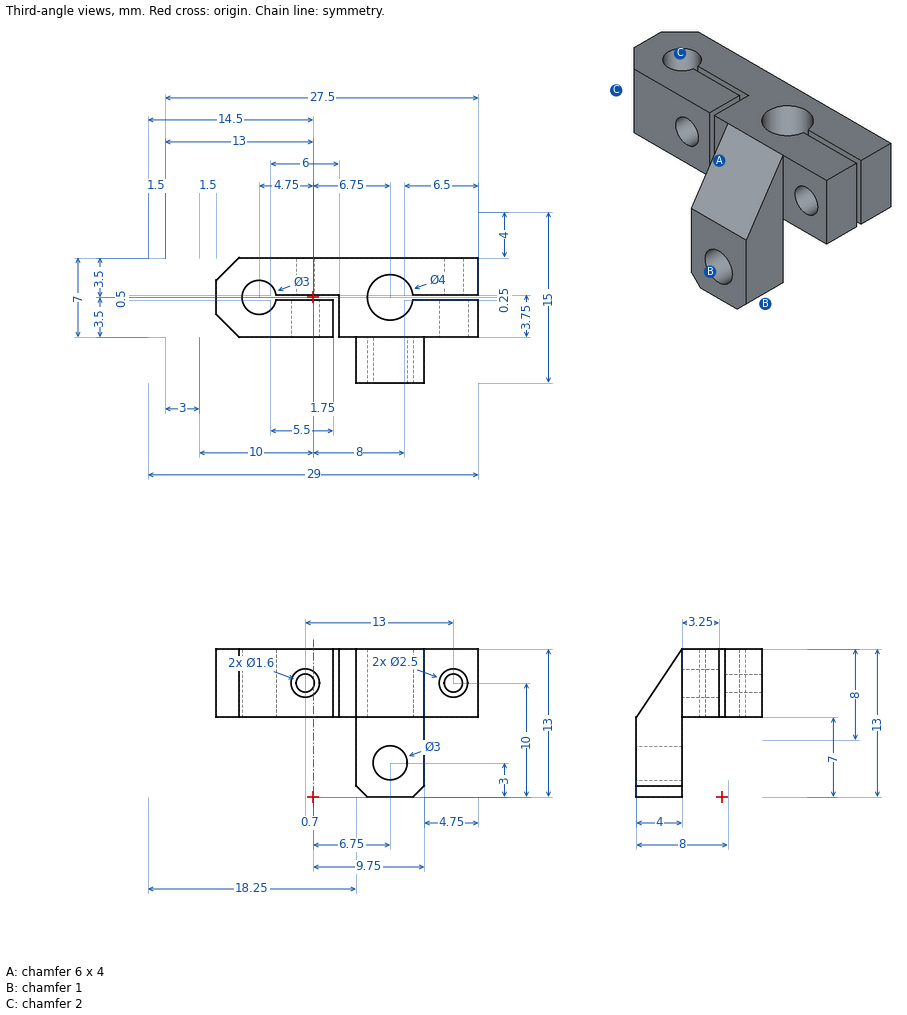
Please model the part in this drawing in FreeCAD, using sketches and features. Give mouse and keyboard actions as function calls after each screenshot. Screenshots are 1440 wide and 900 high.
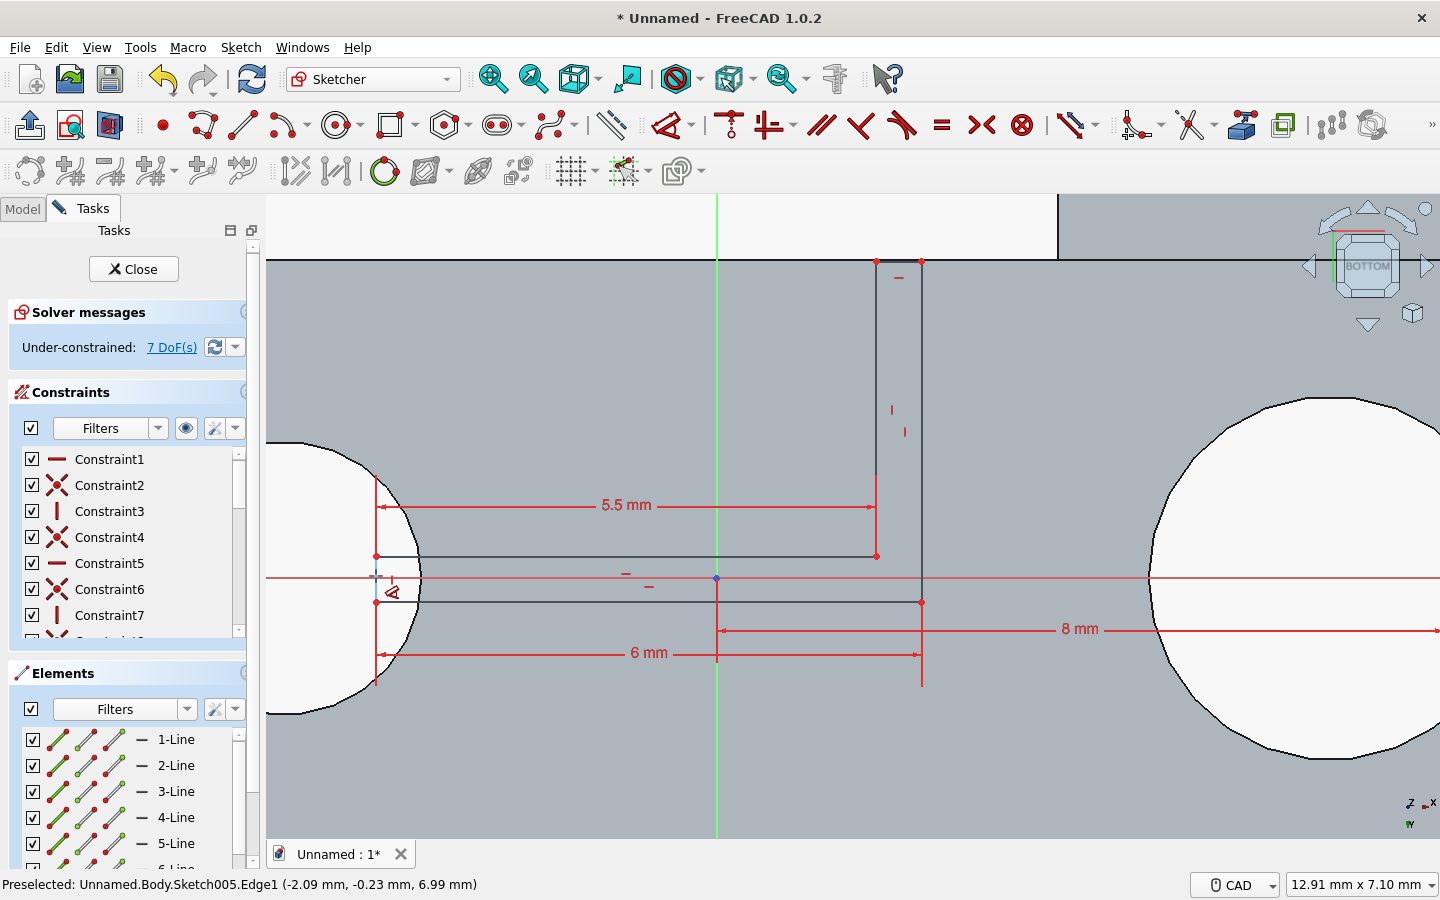
click(376, 575)
click(342, 564)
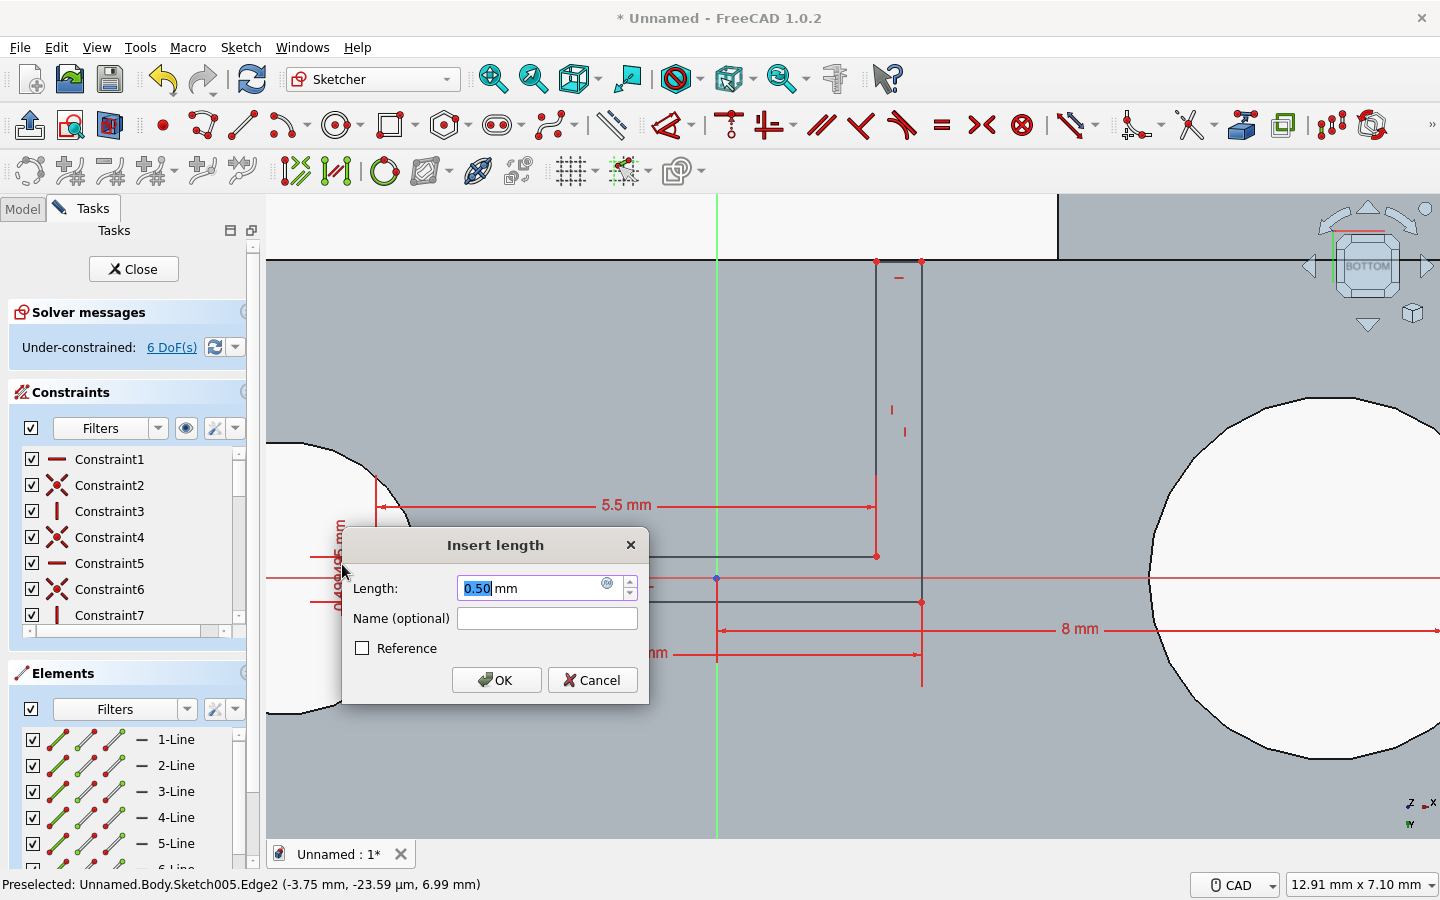
text(0.5)
key(Return)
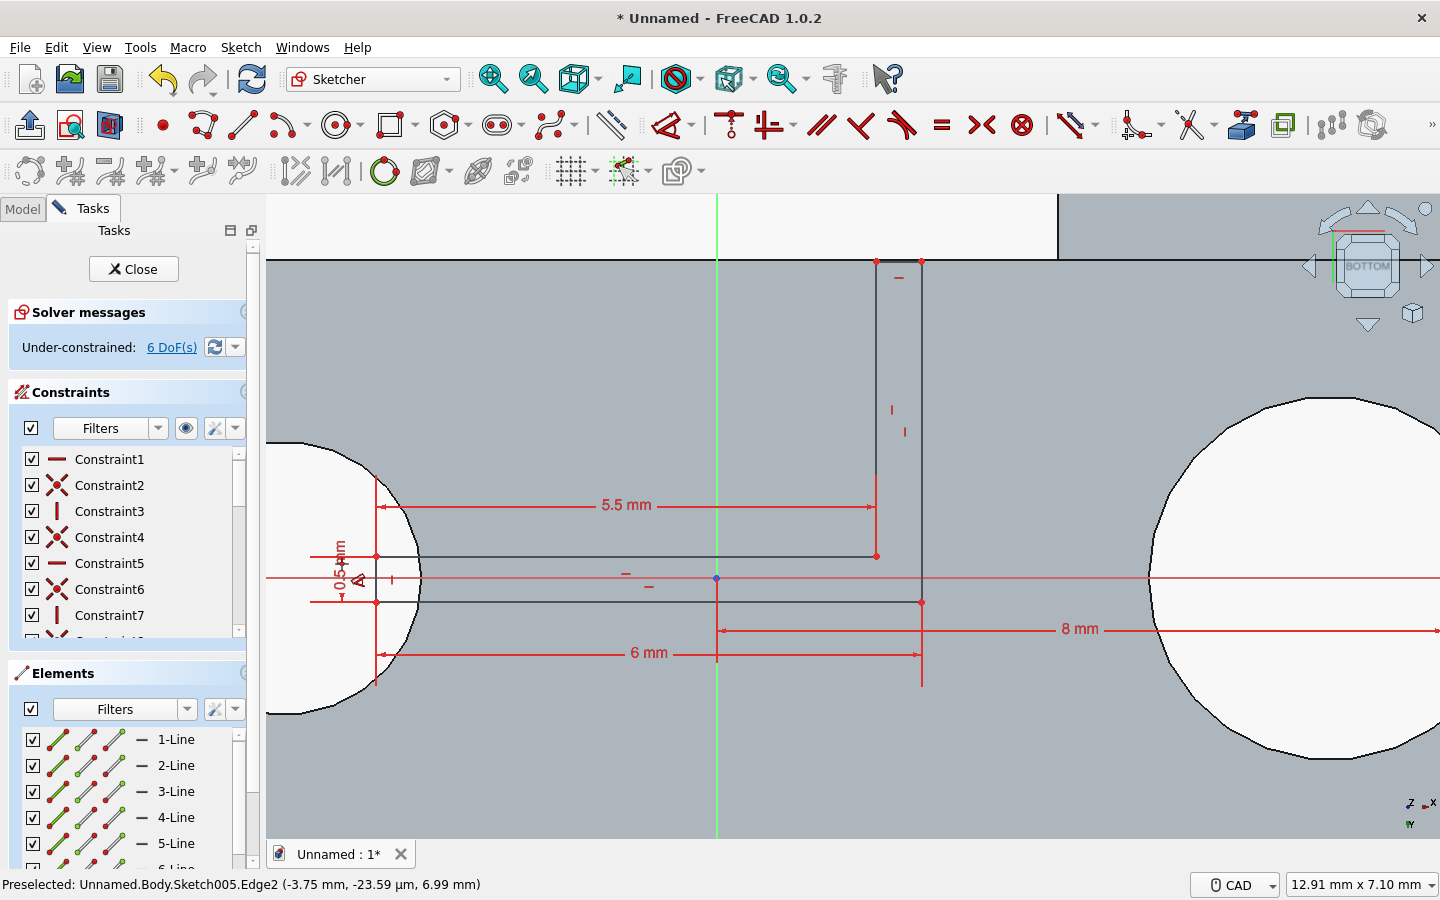
scroll(441, 587, down, 4)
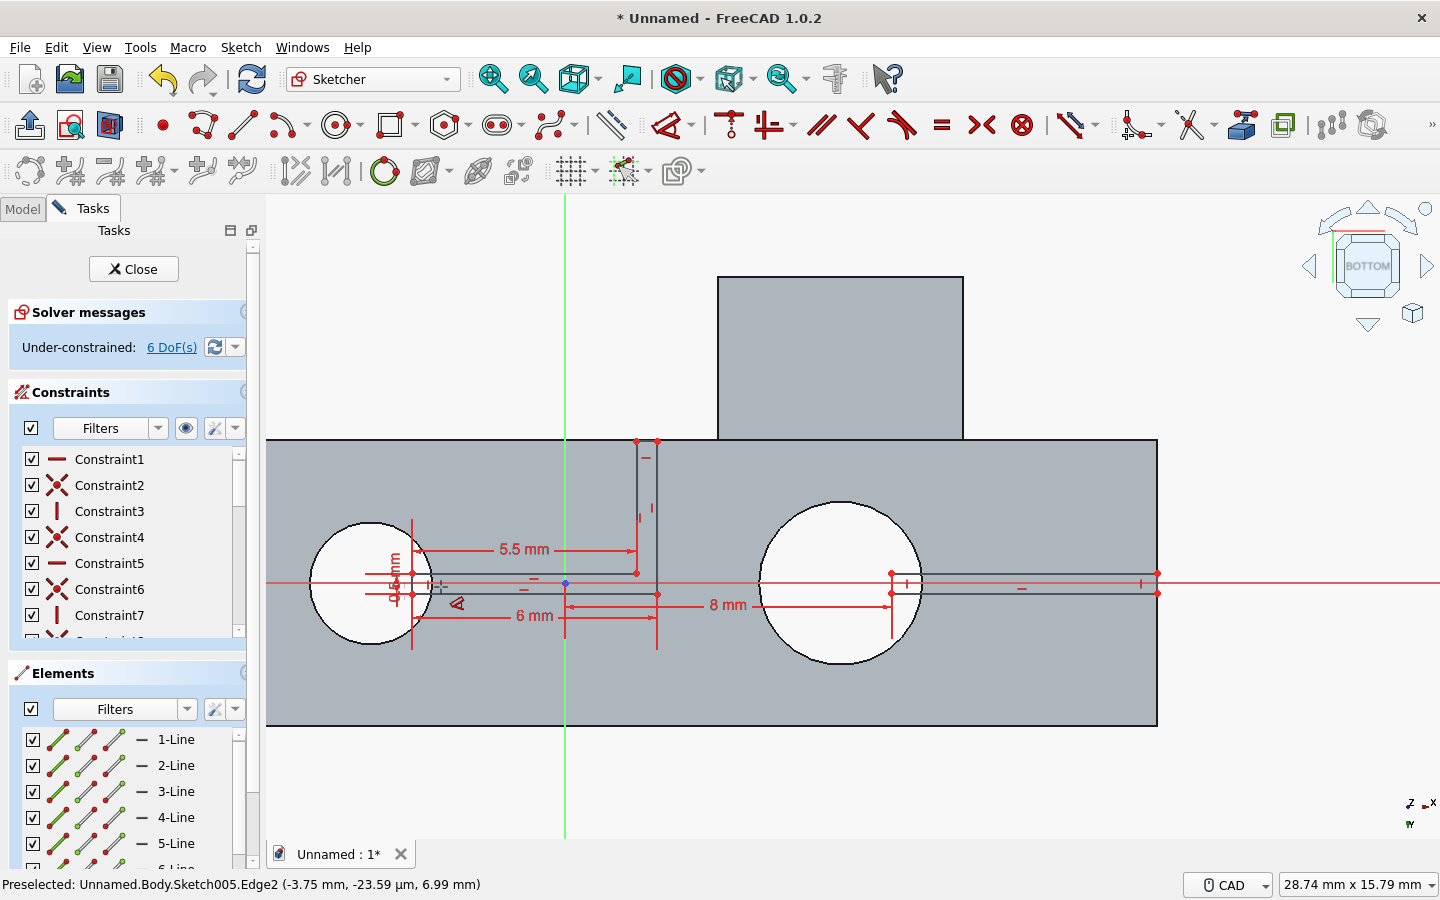
scroll(892, 588, up, 6)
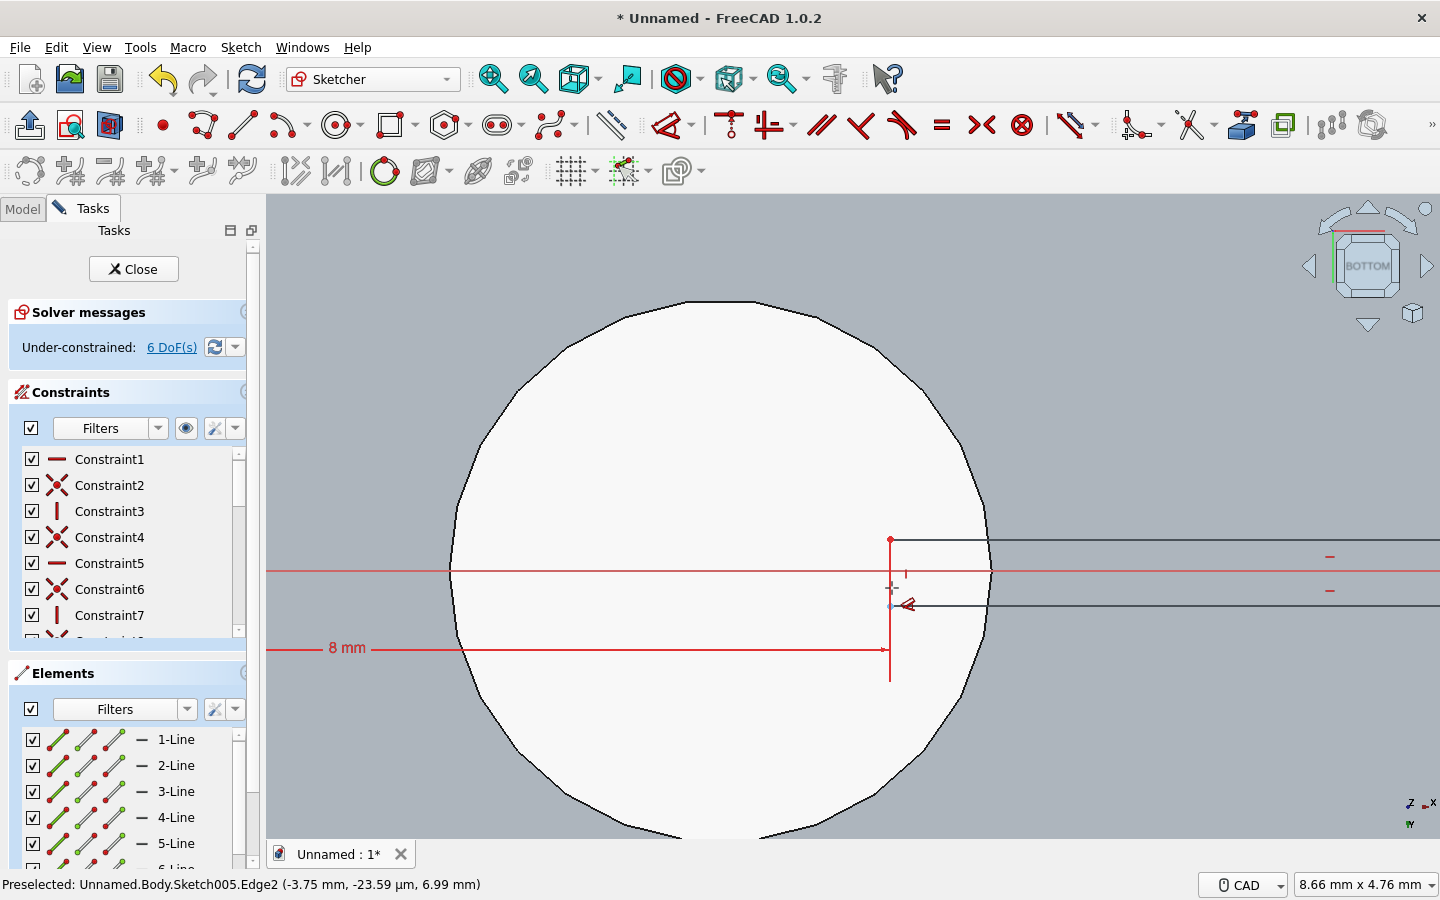
click(890, 586)
click(924, 558)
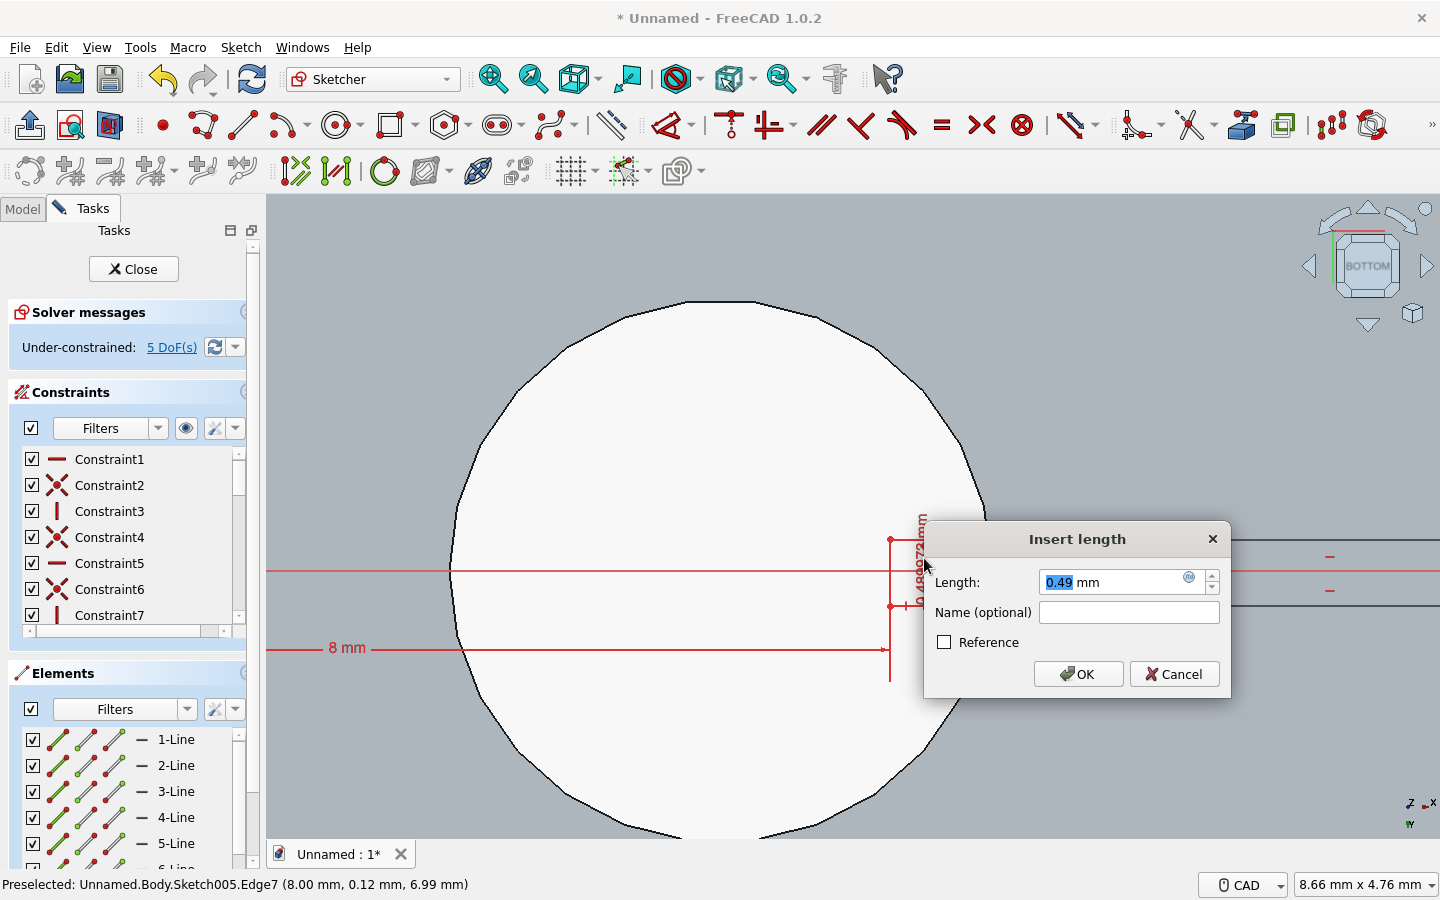
text(0.5)
key(Return)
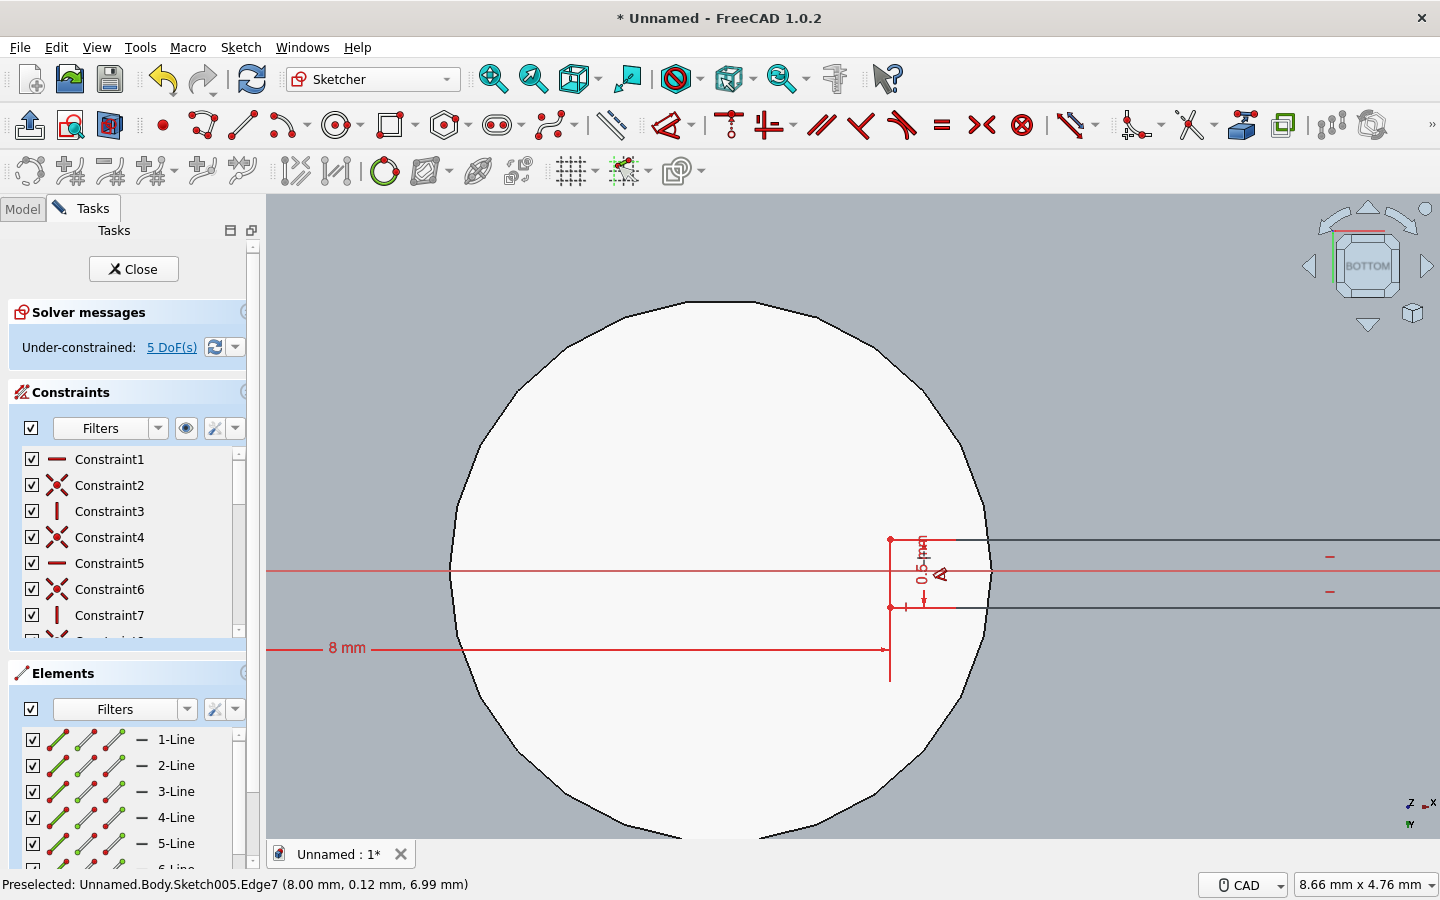
click(1155, 608)
click(1083, 642)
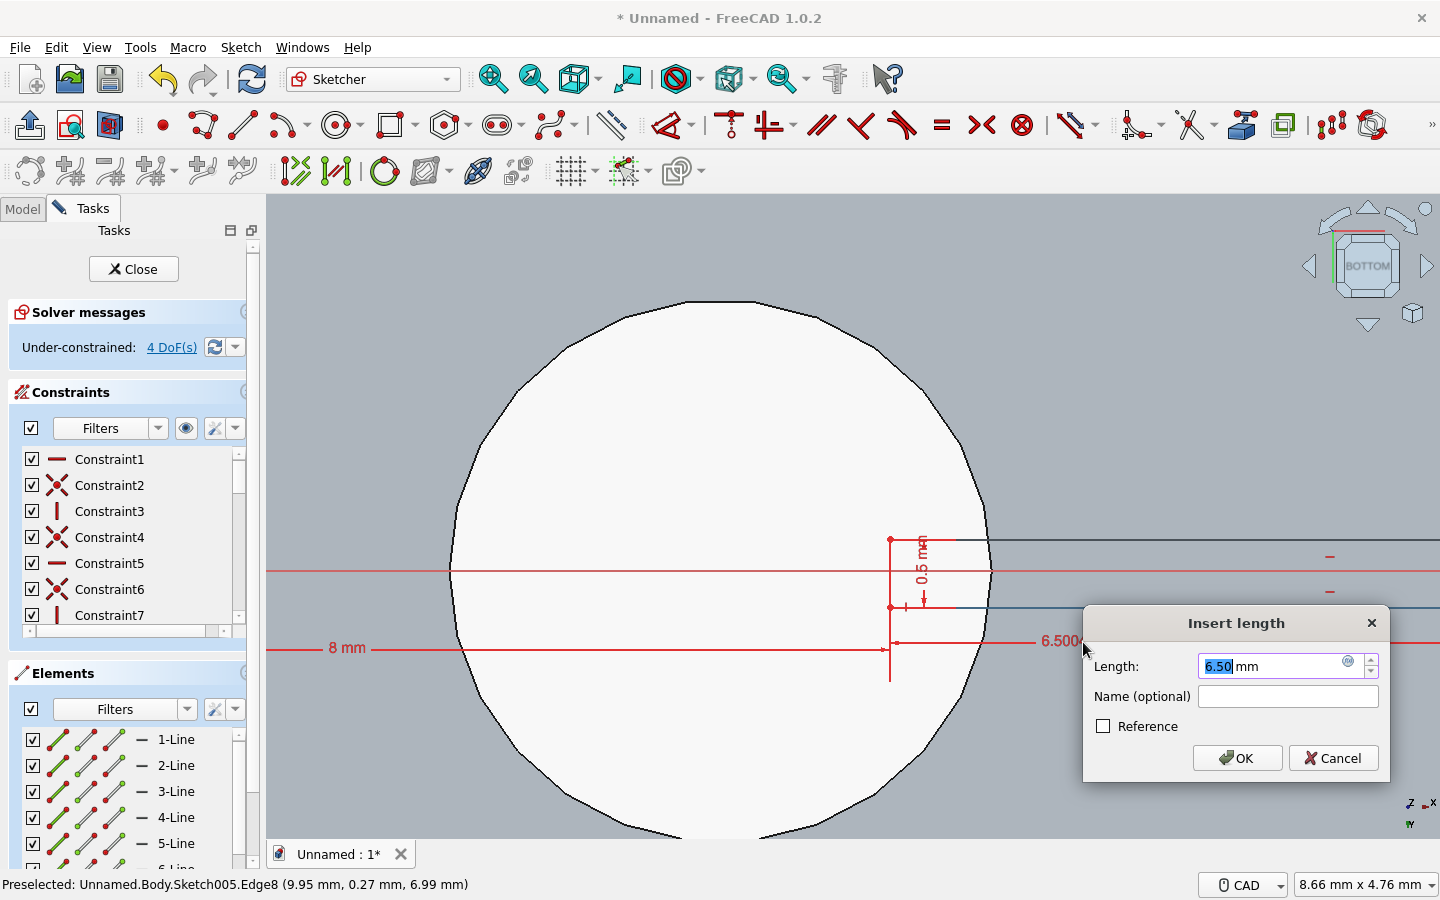
text(6.5)
key(Return)